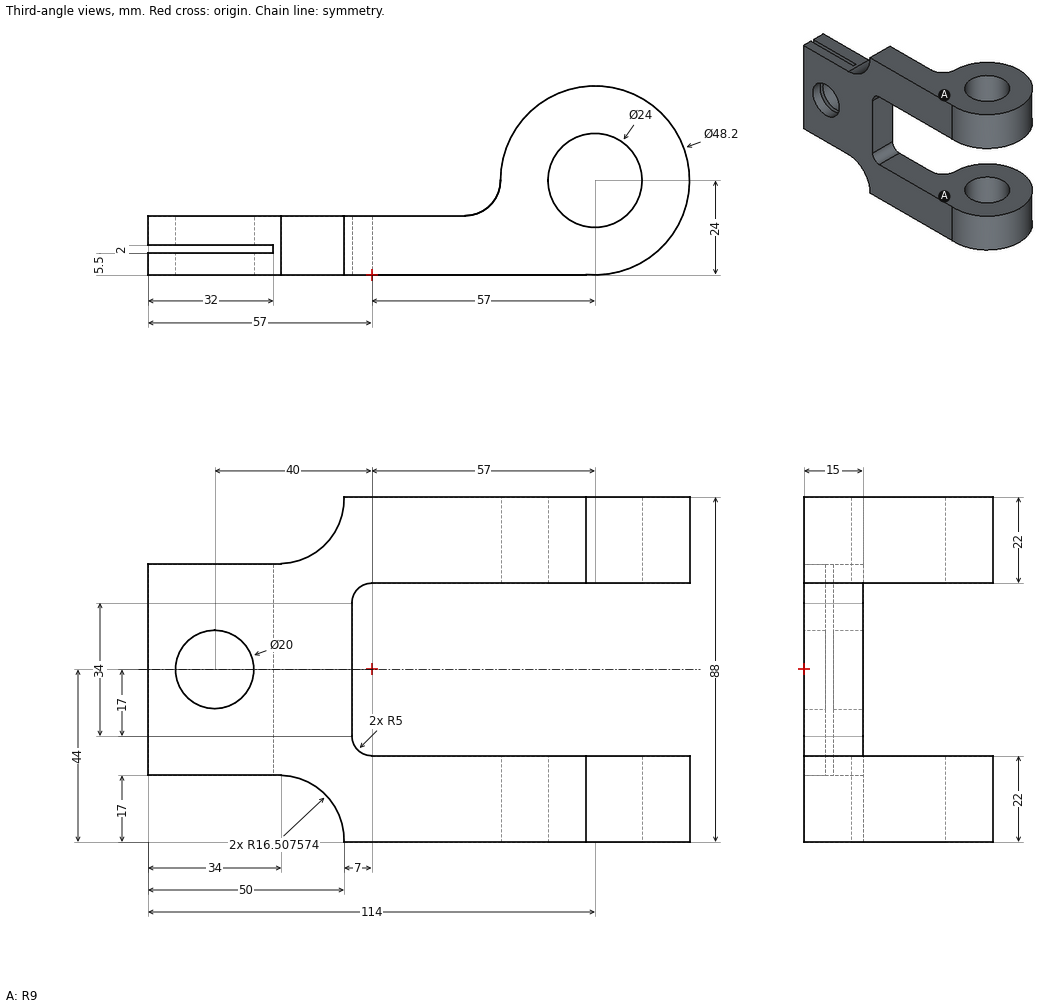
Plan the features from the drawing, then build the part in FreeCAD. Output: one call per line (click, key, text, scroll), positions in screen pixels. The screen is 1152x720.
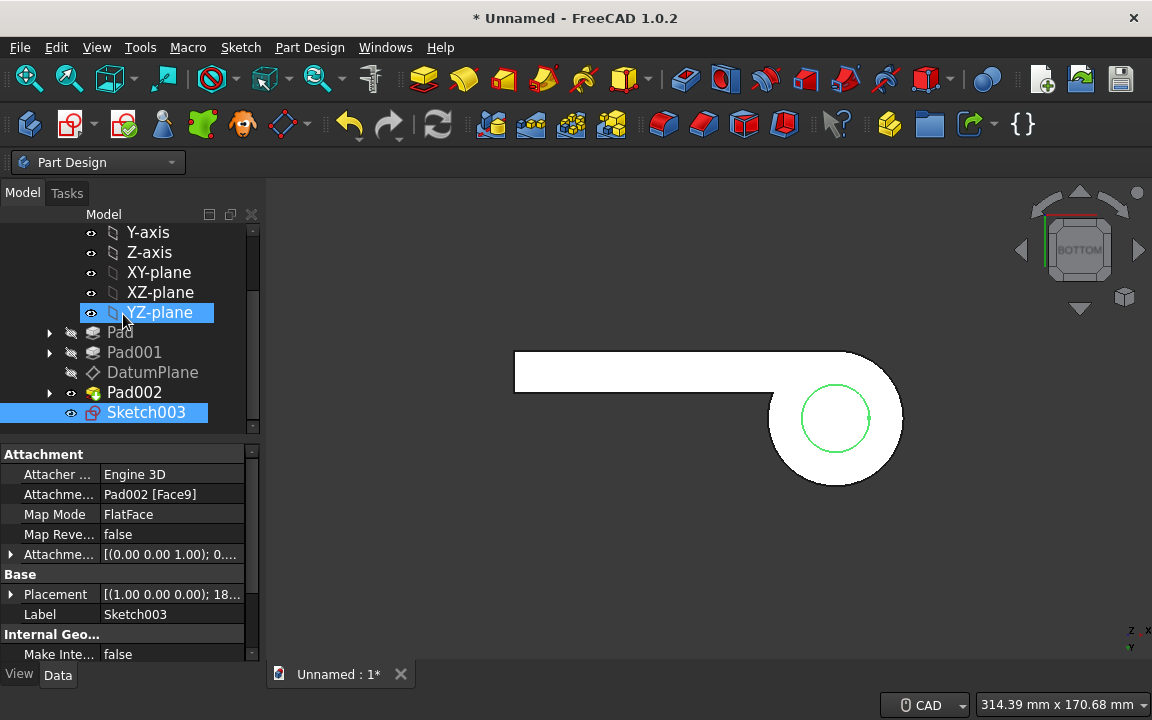
click(686, 80)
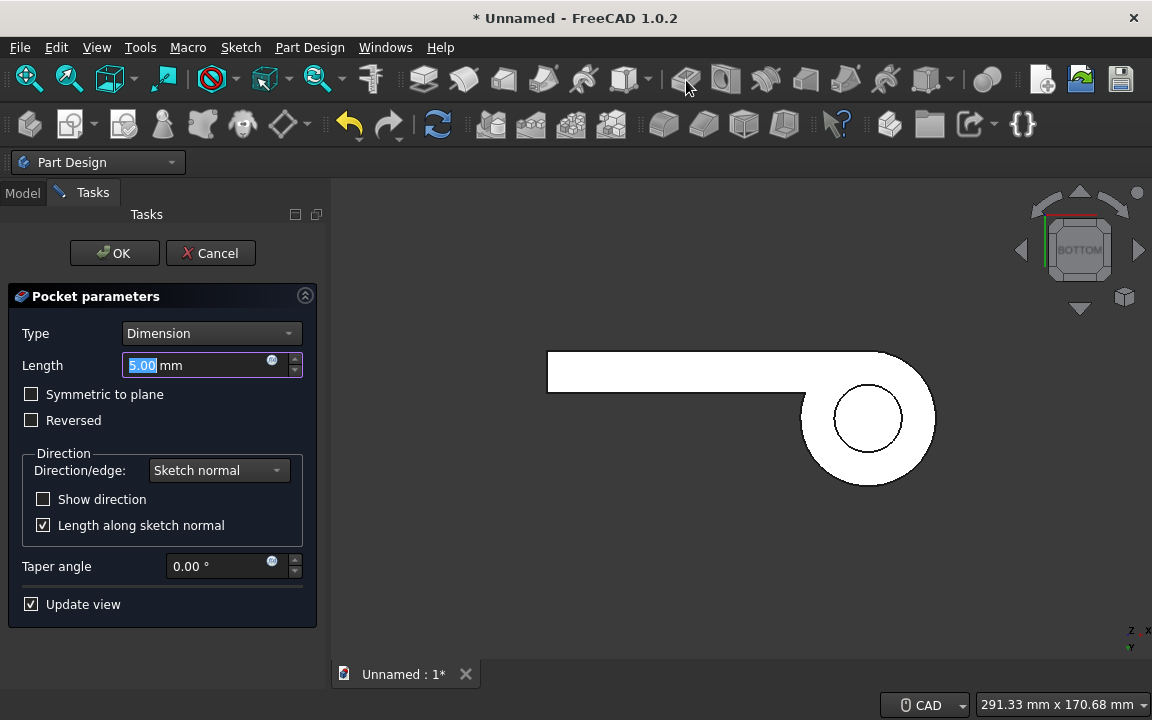
click(212, 334)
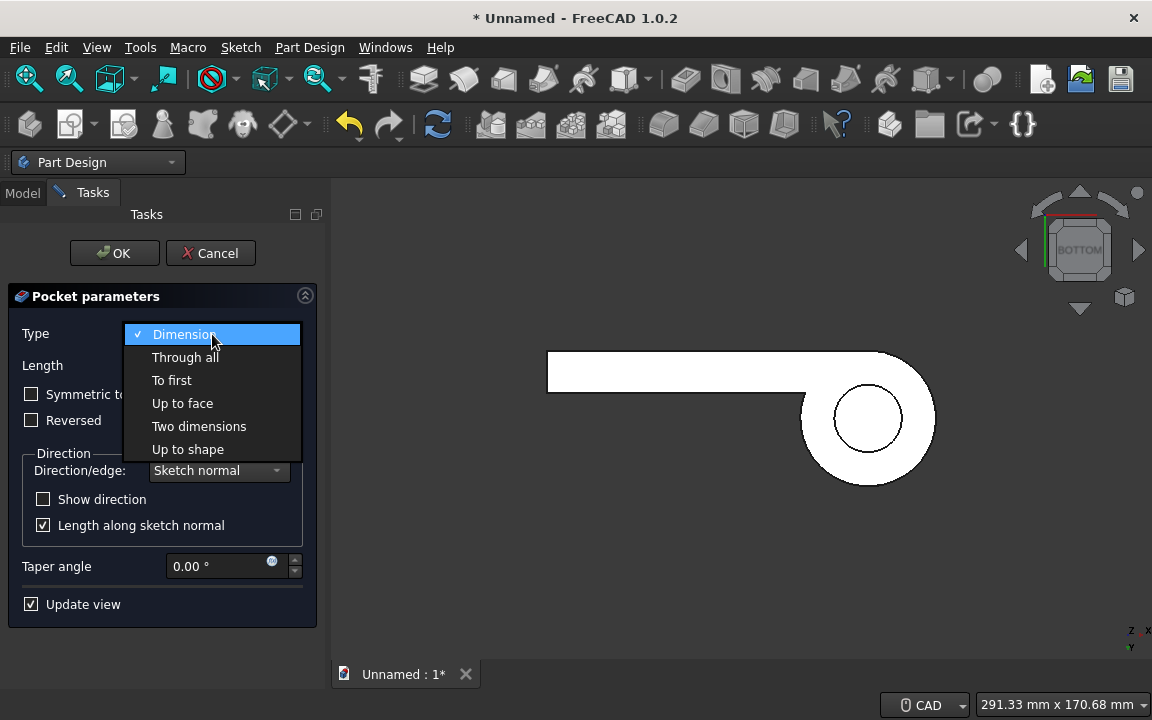
click(212, 358)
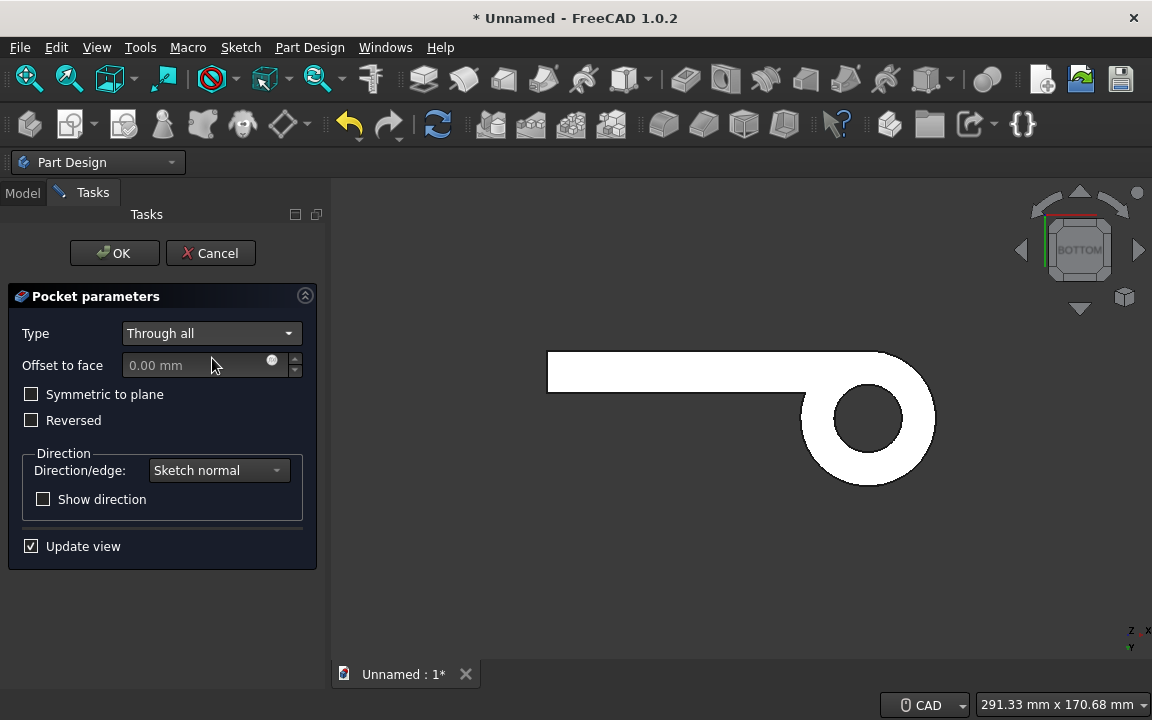
click(115, 253)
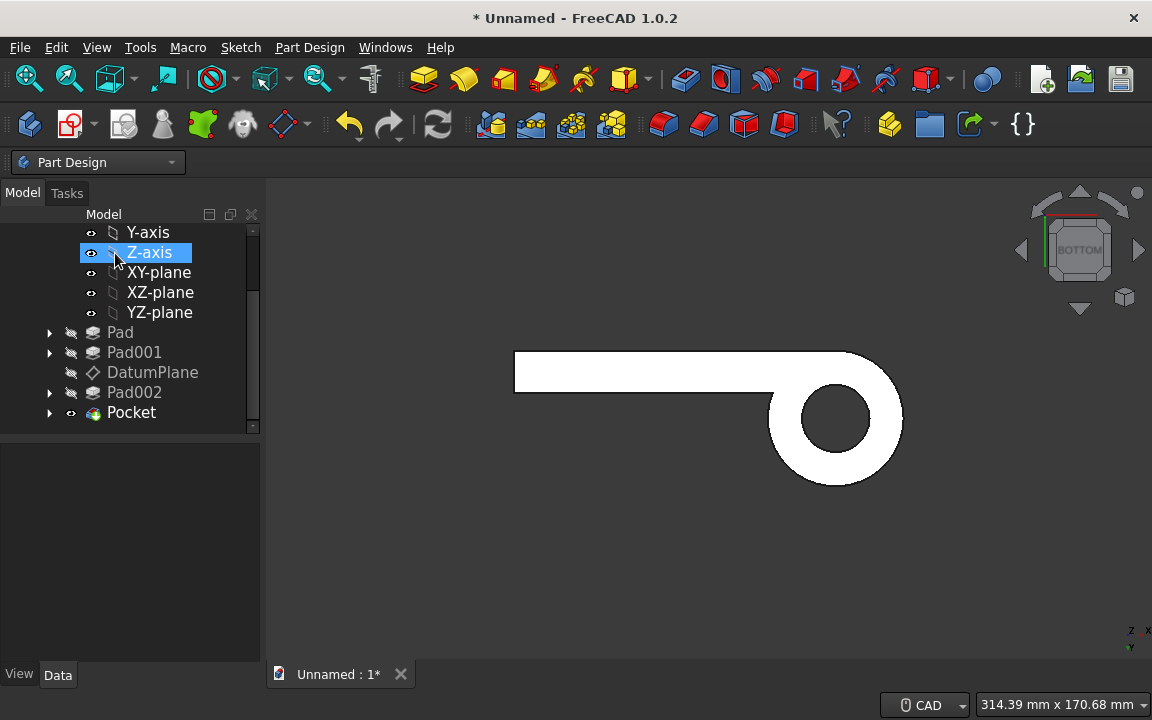
key(v)
key(f)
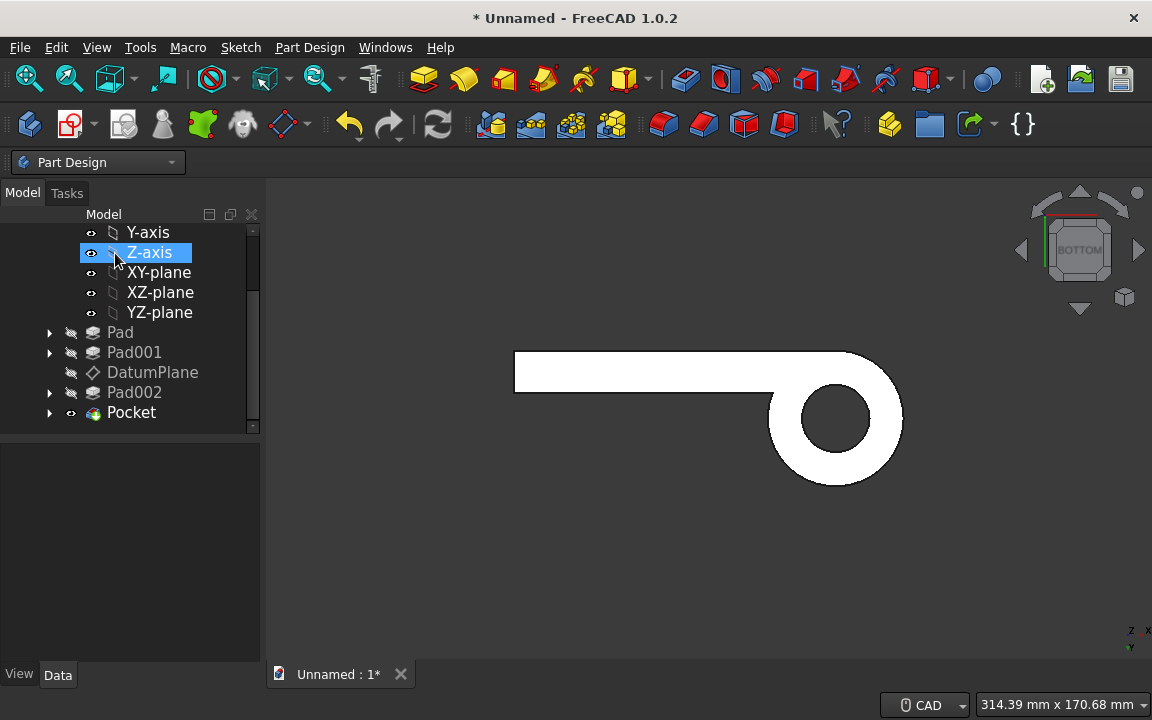
key(0)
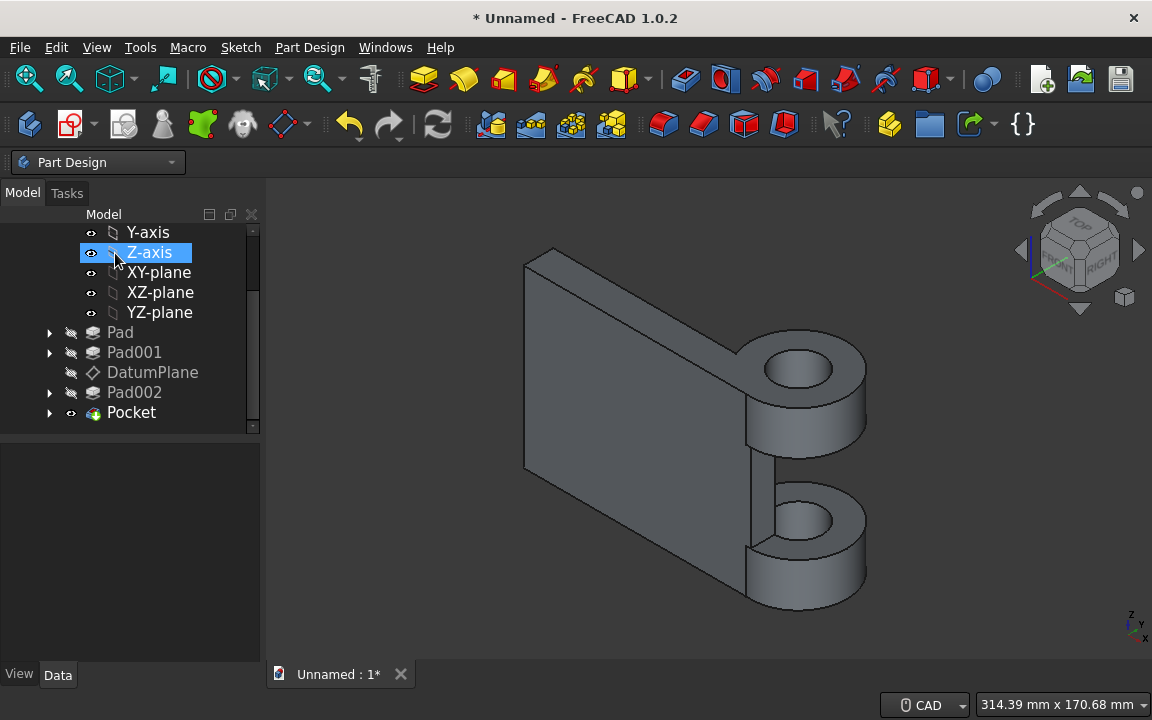
key(2)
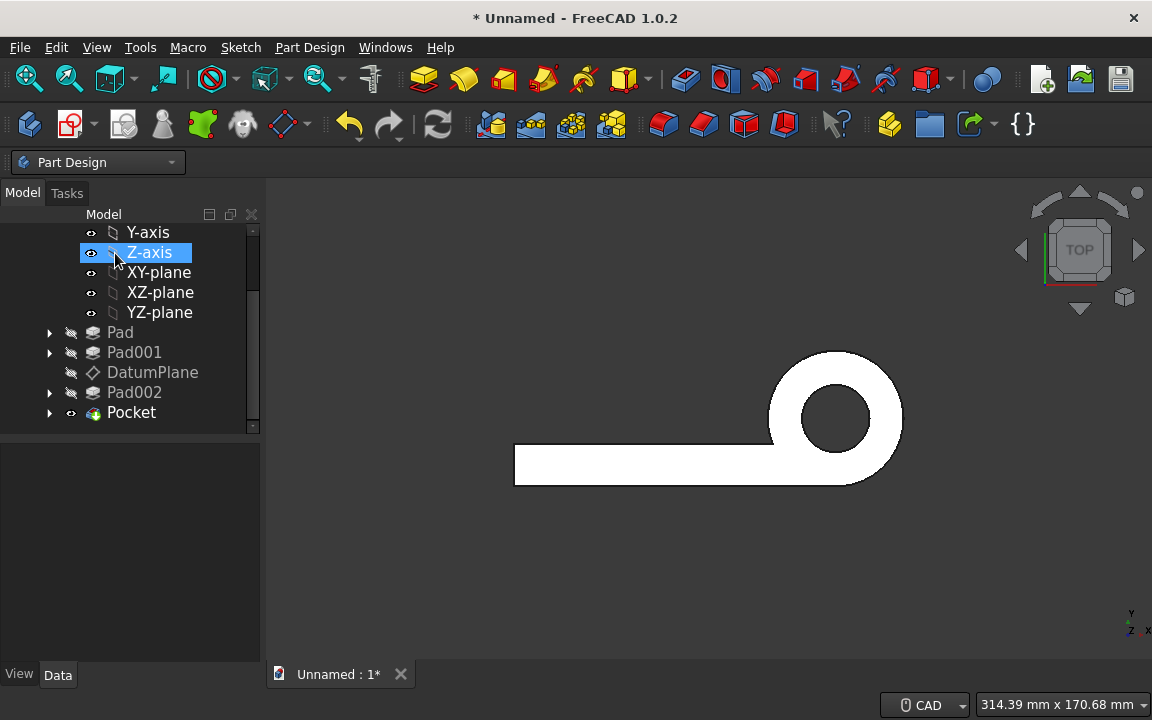
key(v)
key(f)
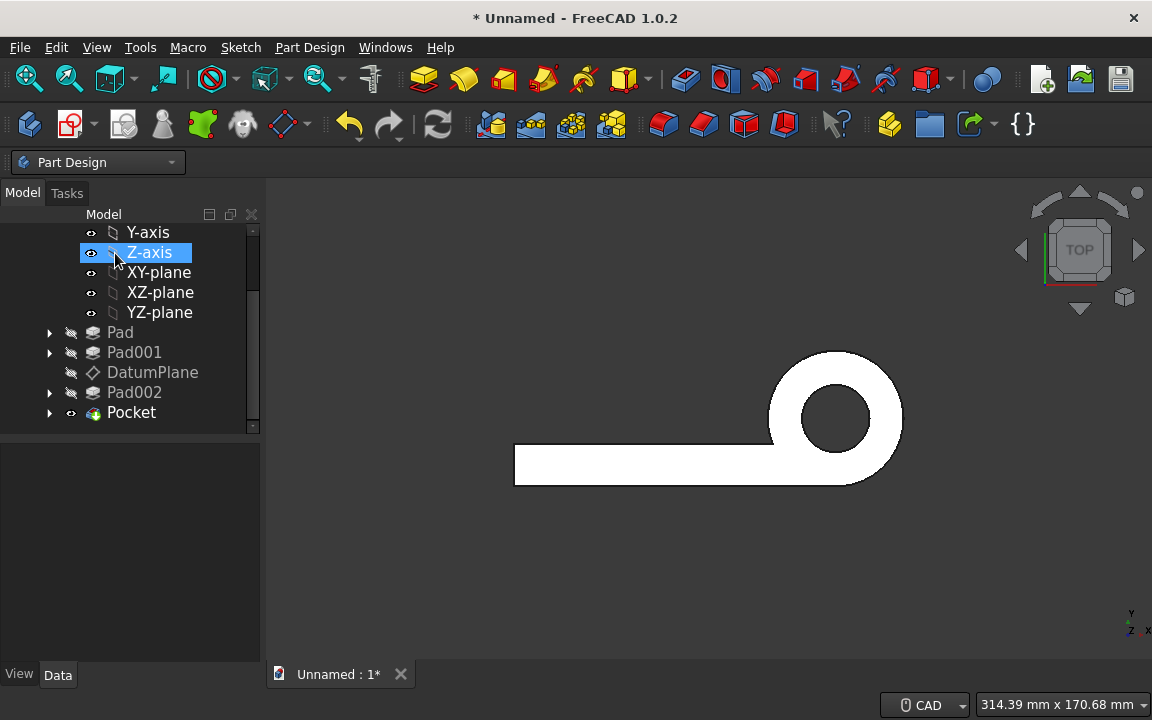
key(1)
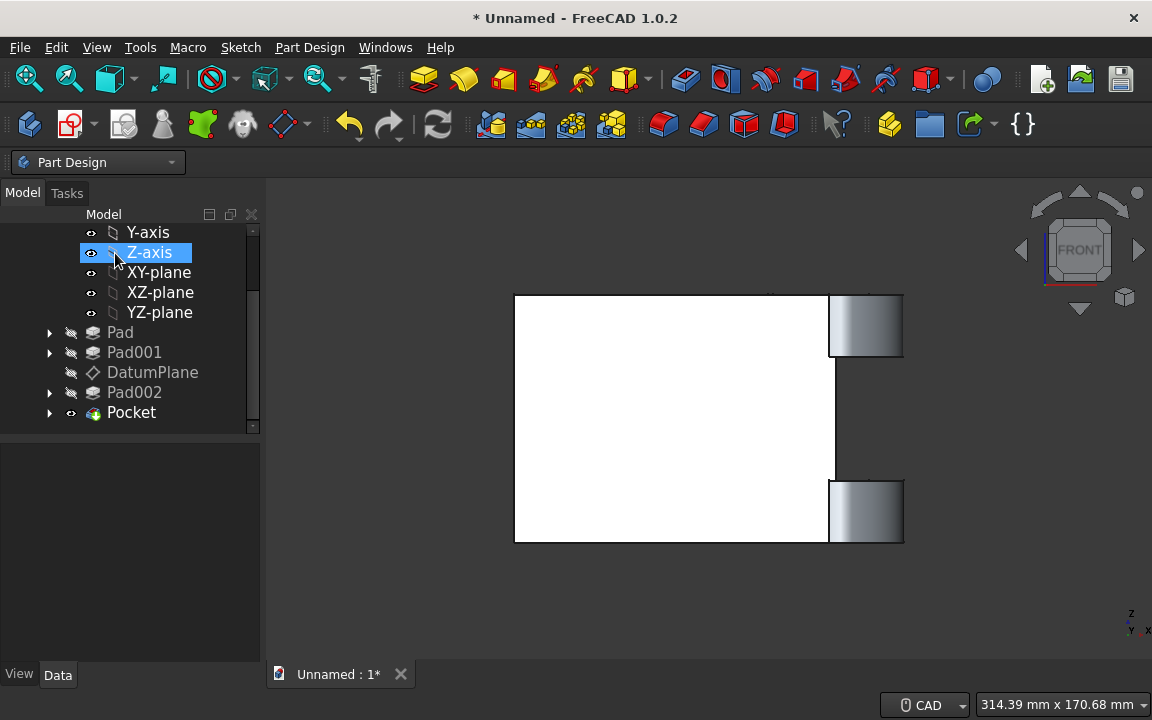
key(3)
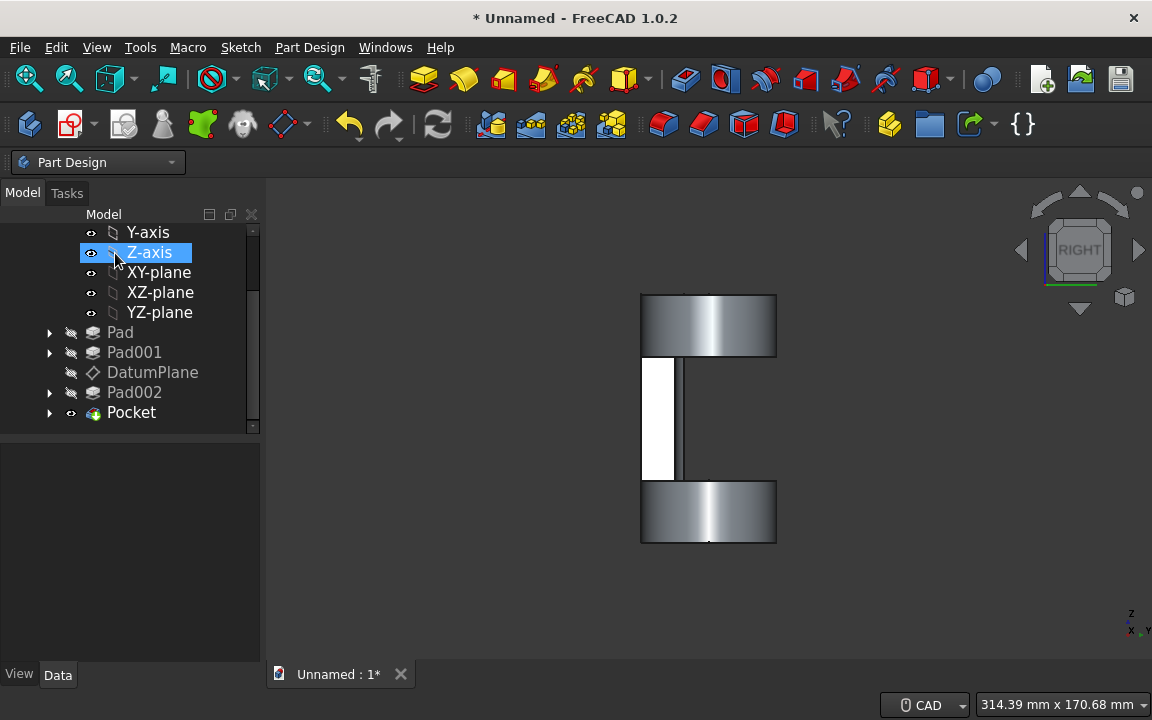
key(5)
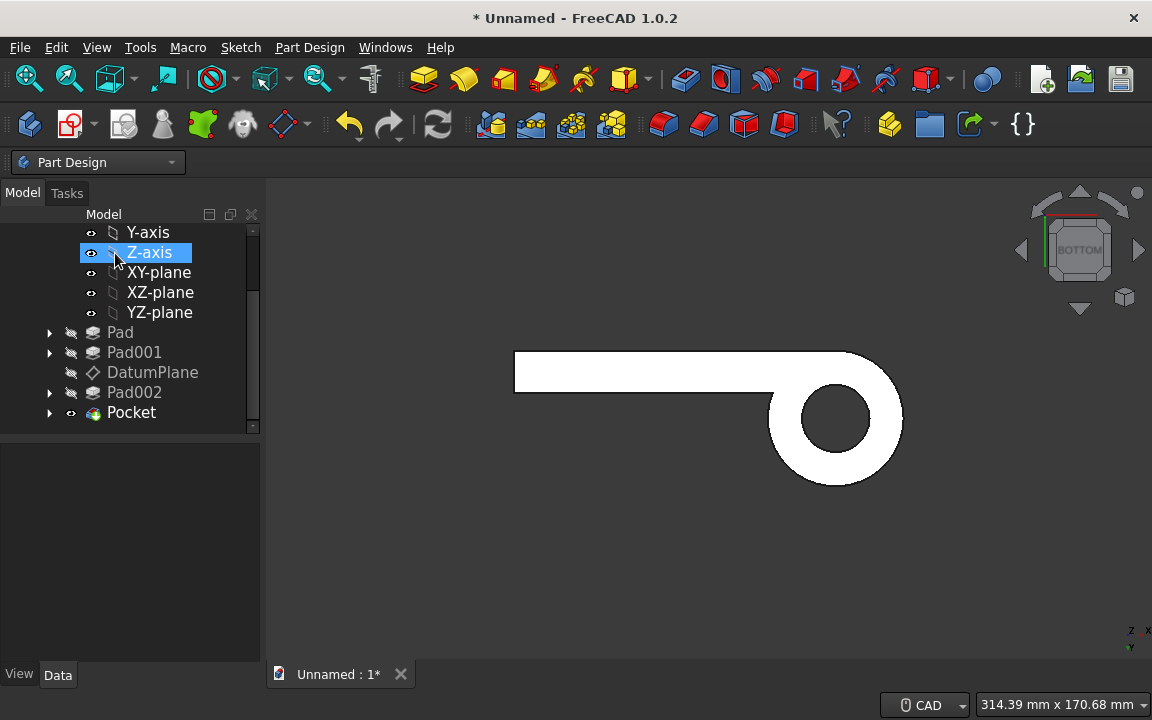
click(30, 80)